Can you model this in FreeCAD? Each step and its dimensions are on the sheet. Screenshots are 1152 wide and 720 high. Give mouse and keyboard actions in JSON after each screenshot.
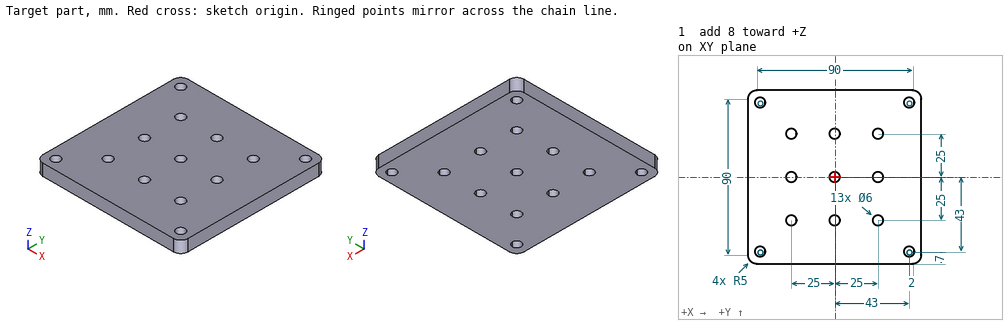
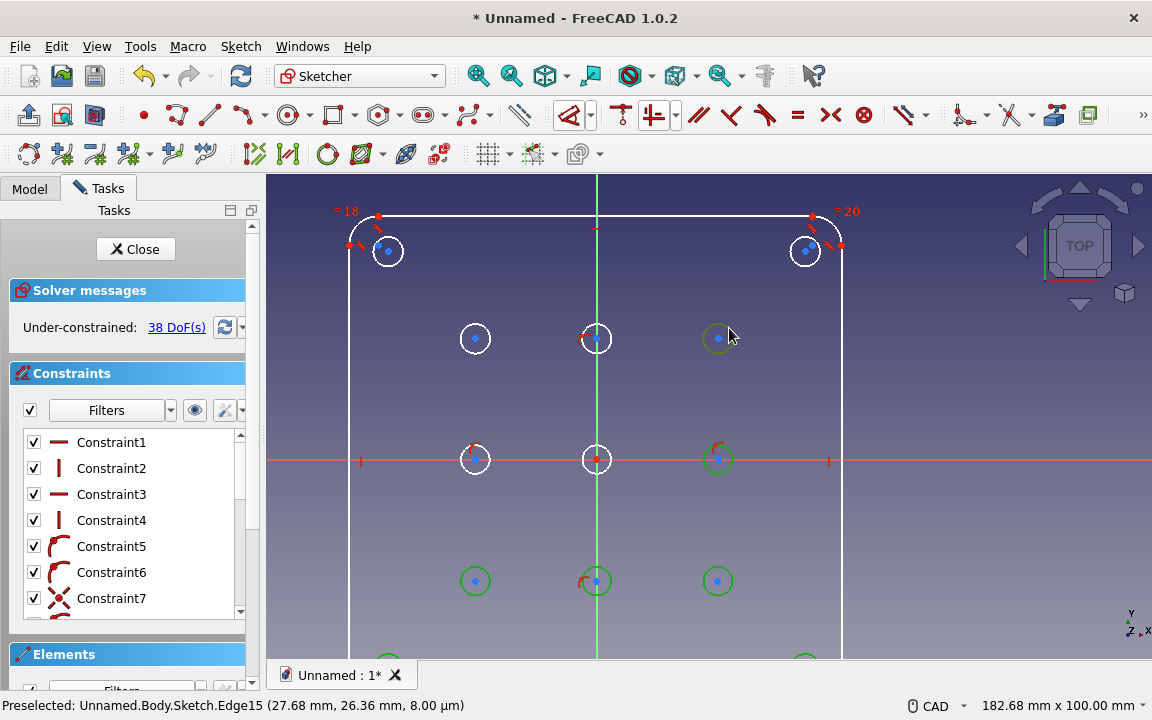
{"action": "left_click", "coordinate": [795, 241]}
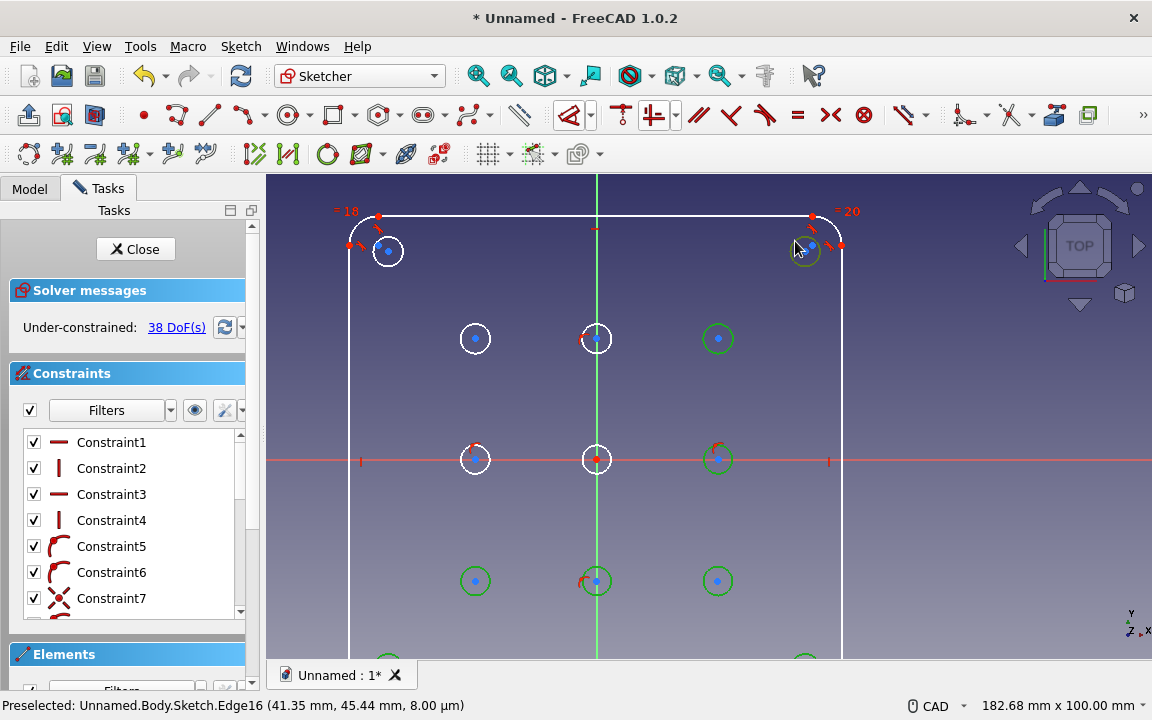
{"action": "scroll", "coordinate": [607, 449], "scroll_direction": "up", "scroll_amount": 2}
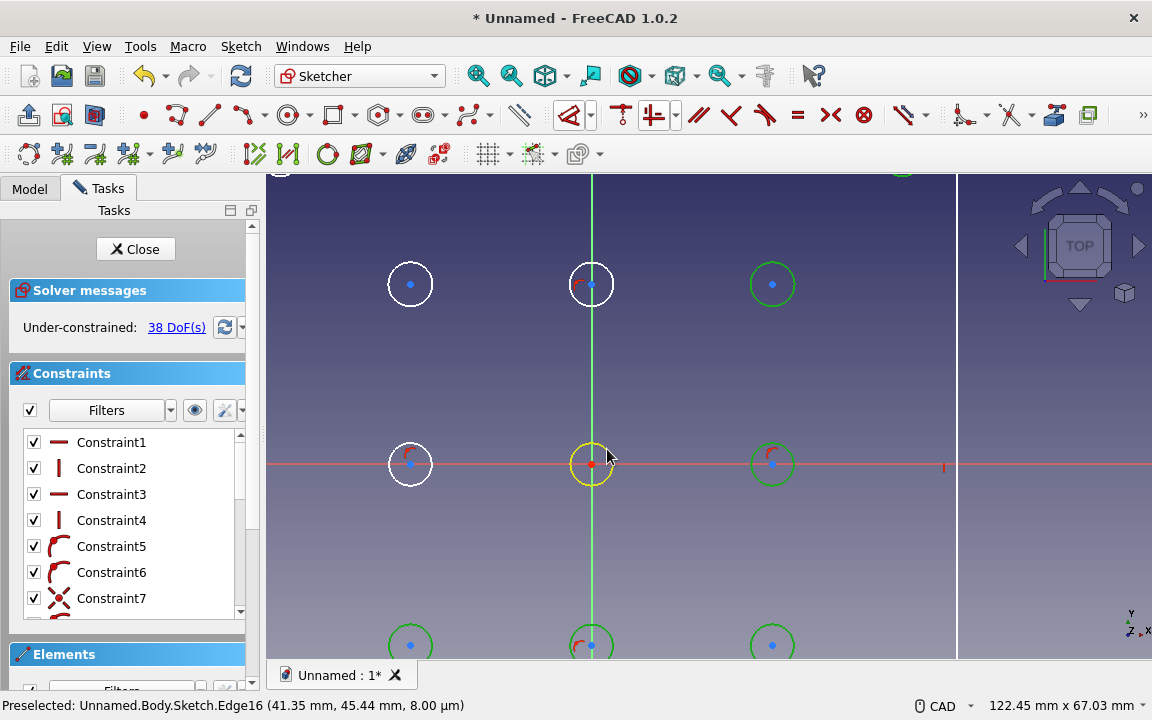
{"action": "left_click", "coordinate": [606, 449]}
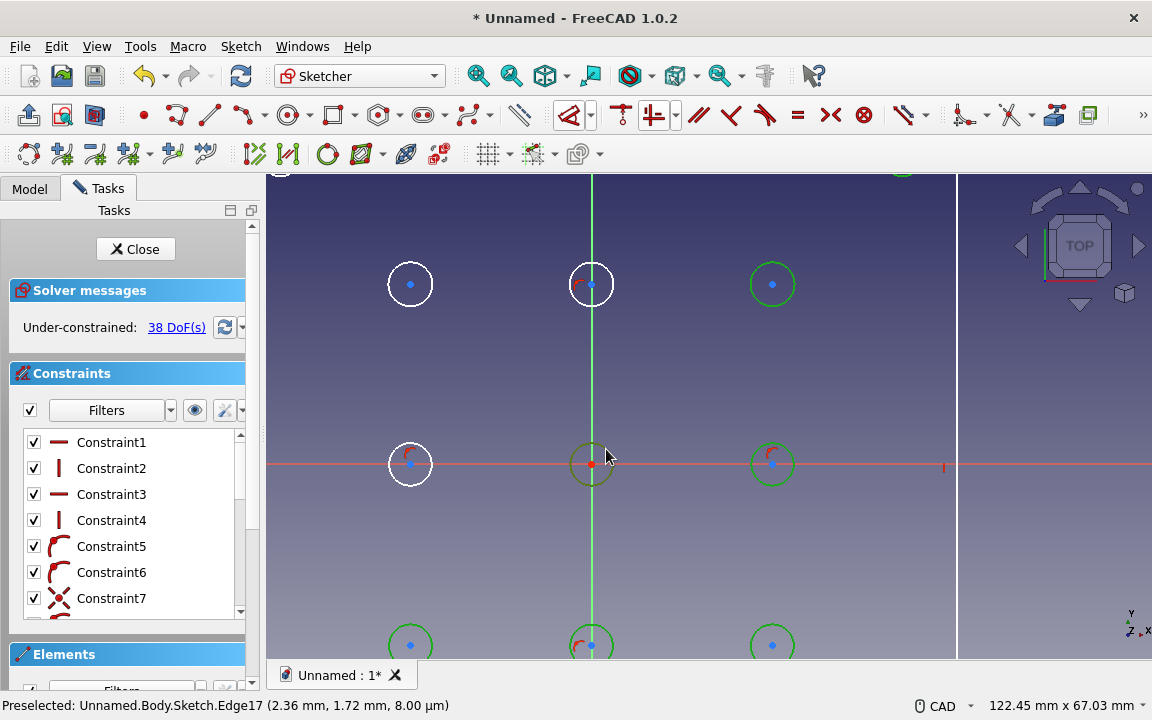
{"action": "left_click", "coordinate": [425, 449]}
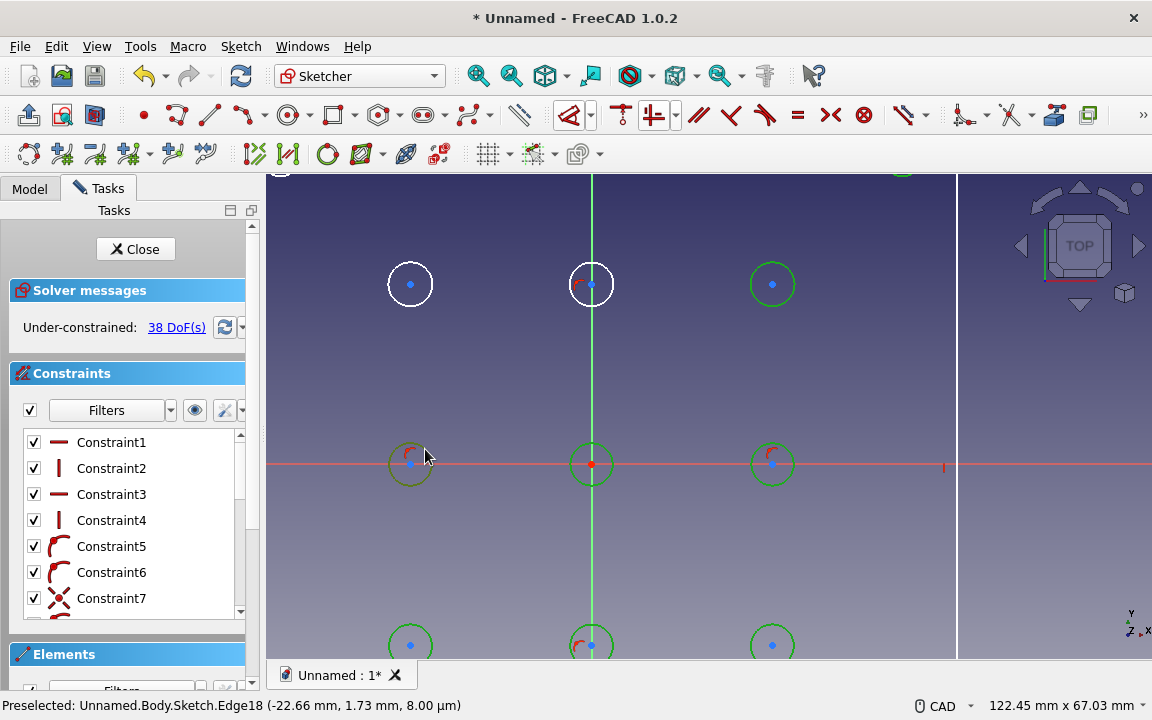
{"action": "left_click", "coordinate": [607, 269]}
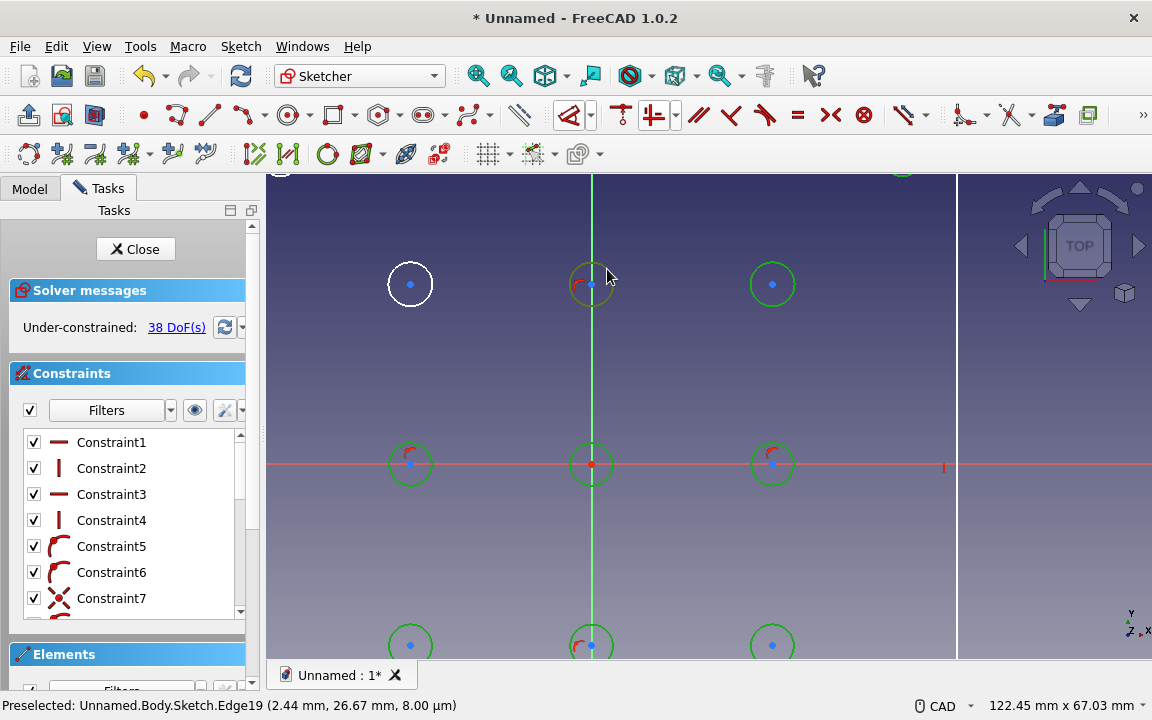
{"action": "left_click", "coordinate": [426, 269]}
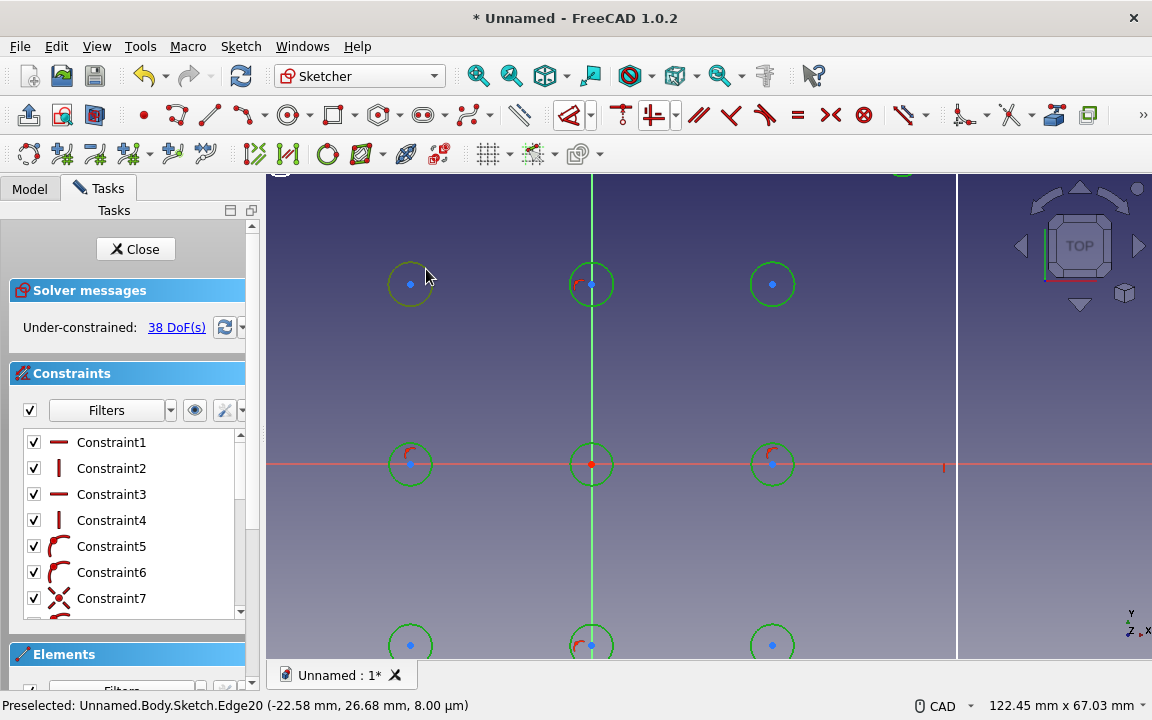
{"action": "scroll", "coordinate": [680, 377], "scroll_direction": "down", "scroll_amount": 4}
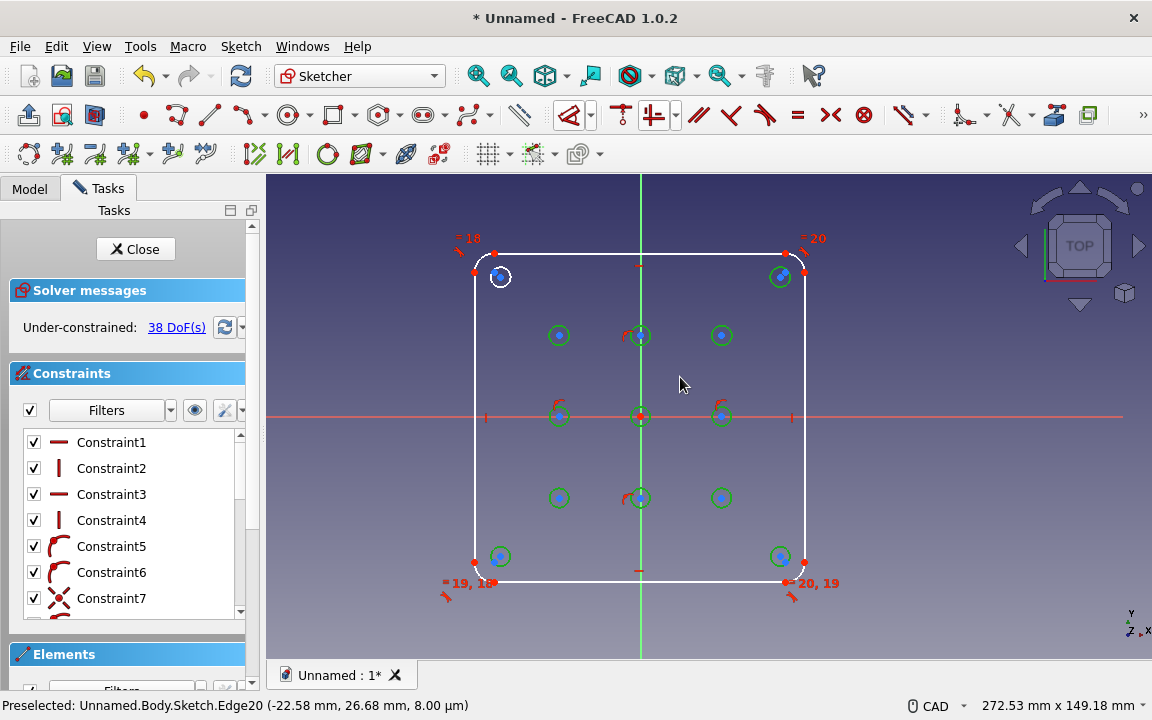
{"action": "scroll", "coordinate": [508, 270], "scroll_direction": "up", "scroll_amount": 2}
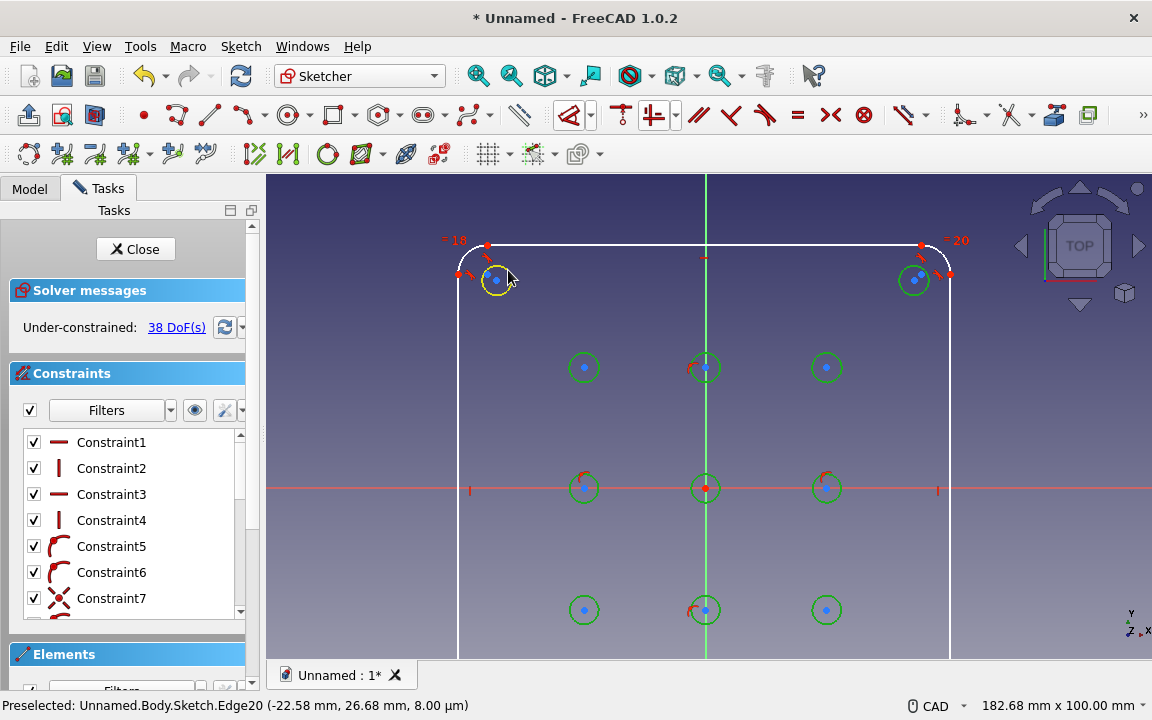
{"action": "left_click", "coordinate": [507, 270]}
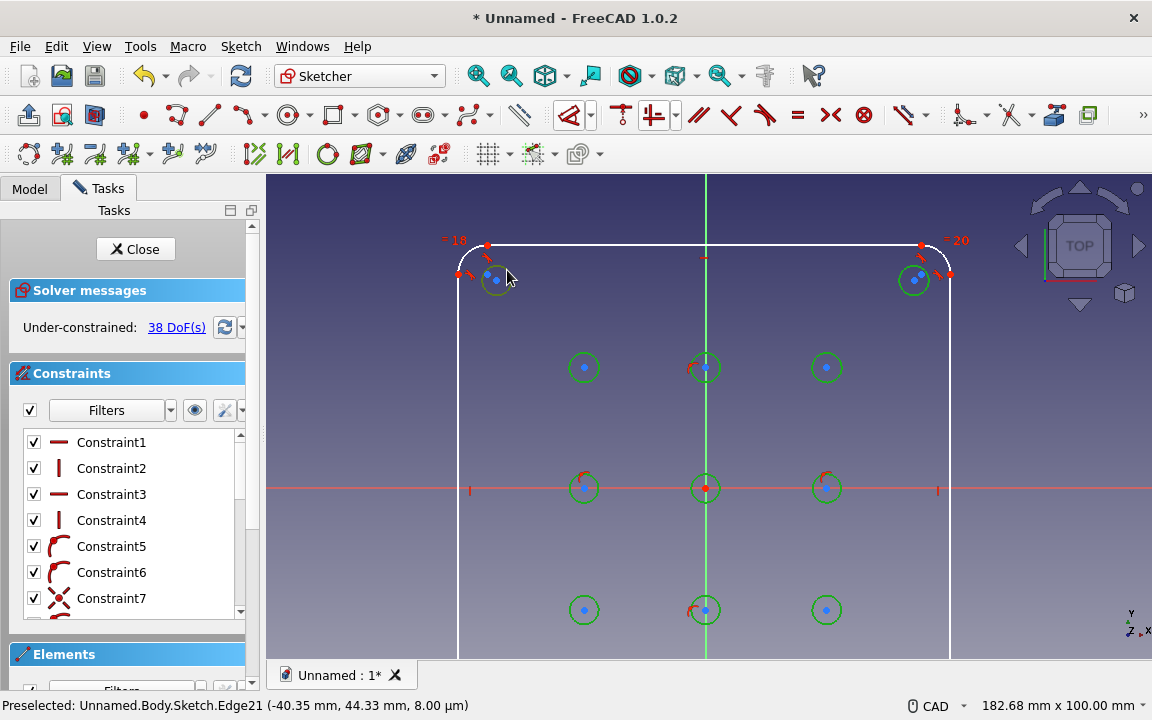
{"action": "left_click", "coordinate": [798, 116]}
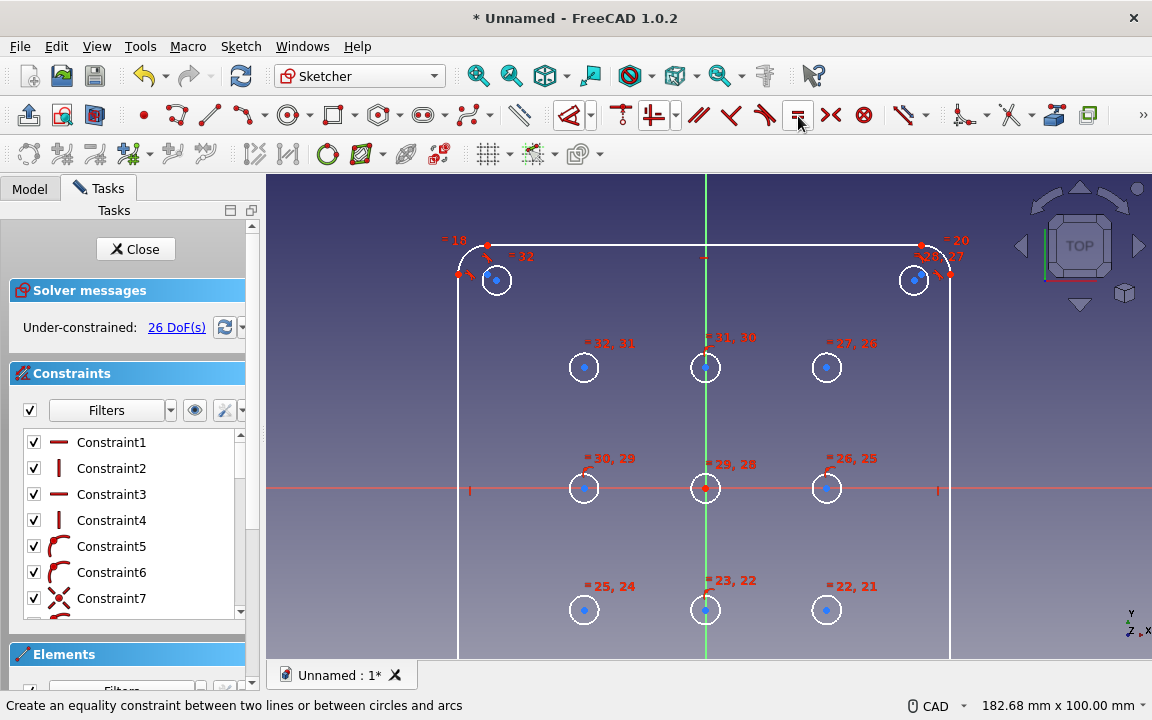
{"action": "left_click", "coordinate": [827, 610]}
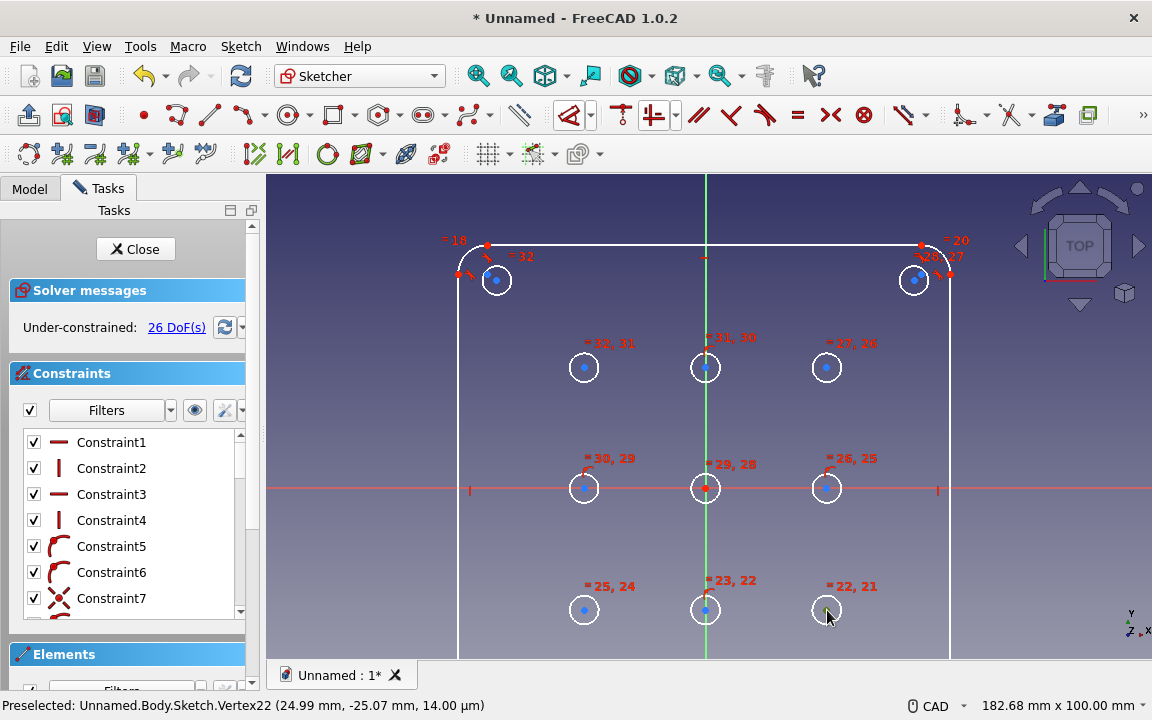
{"action": "left_click", "coordinate": [706, 610]}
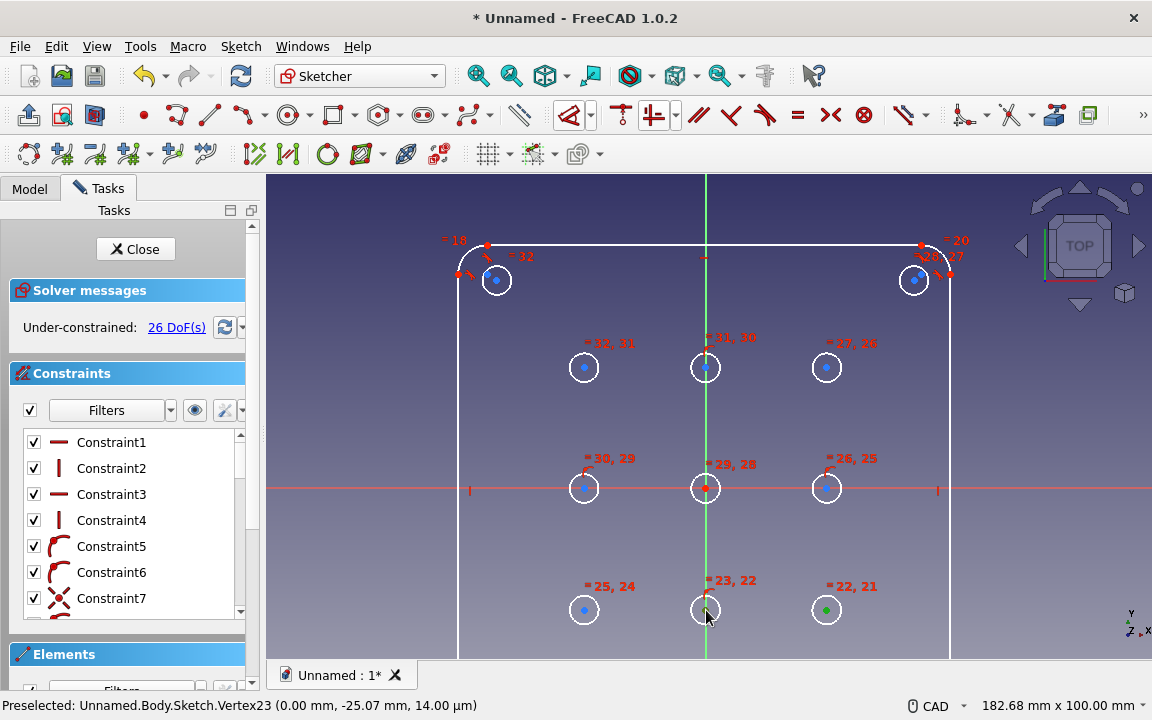
{"action": "left_click", "coordinate": [676, 116]}